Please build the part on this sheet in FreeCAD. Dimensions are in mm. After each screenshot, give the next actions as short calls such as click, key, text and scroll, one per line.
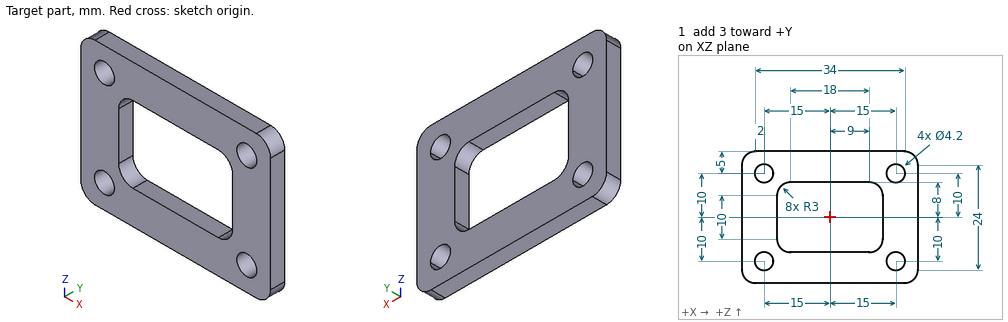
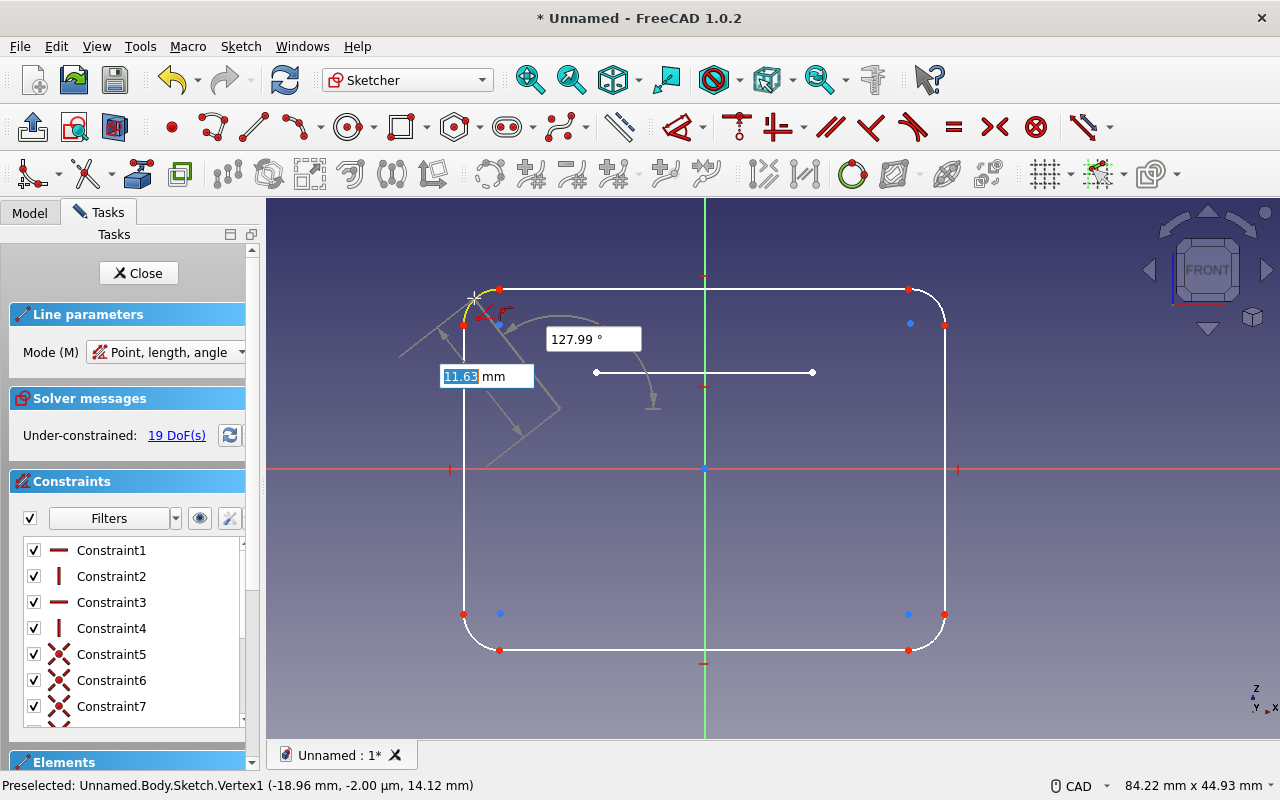
click(560, 529)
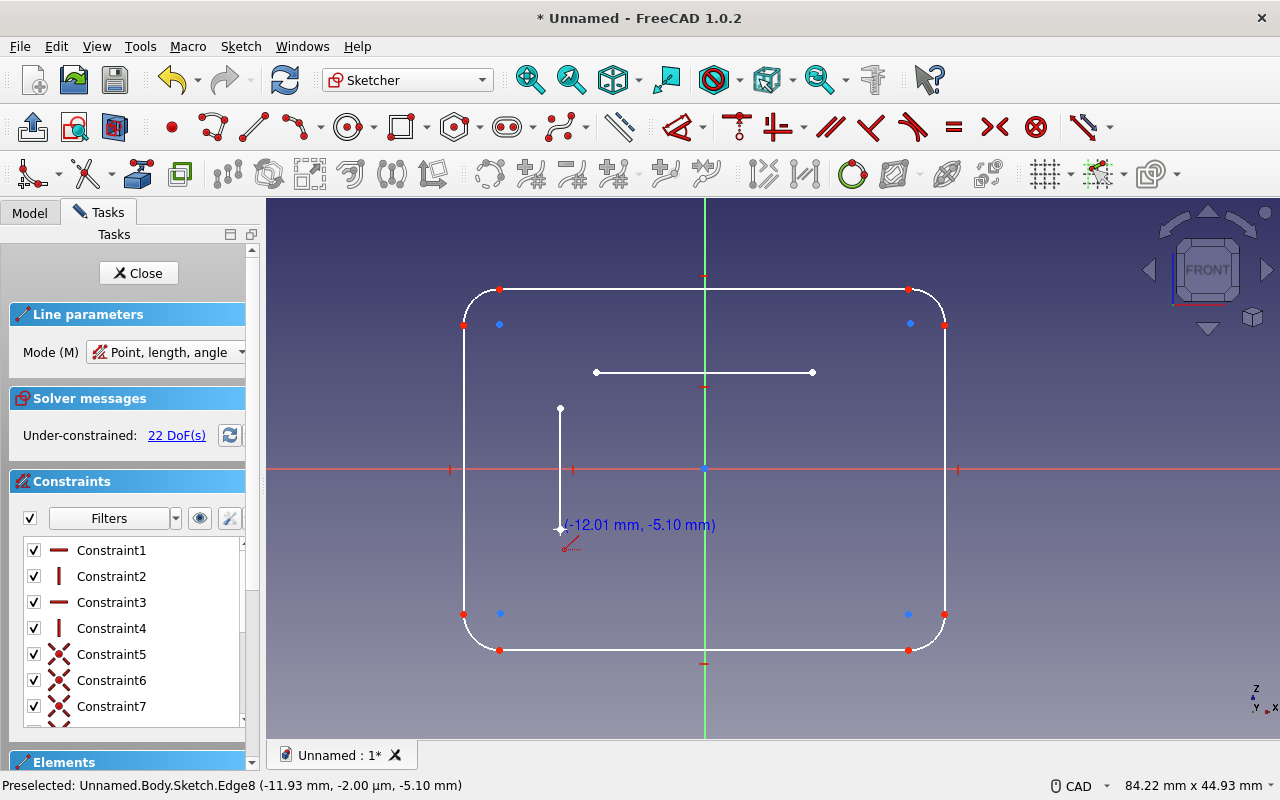
click(596, 565)
click(813, 565)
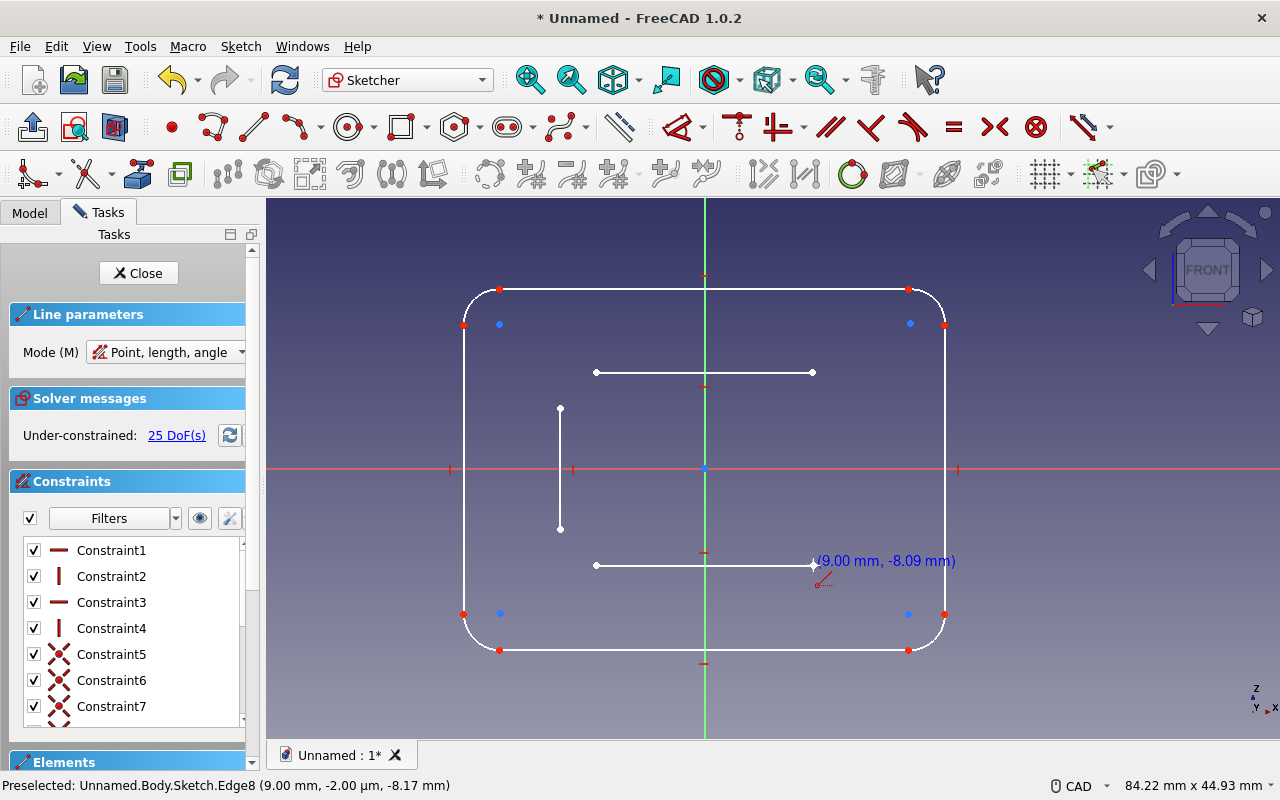
click(849, 529)
click(849, 408)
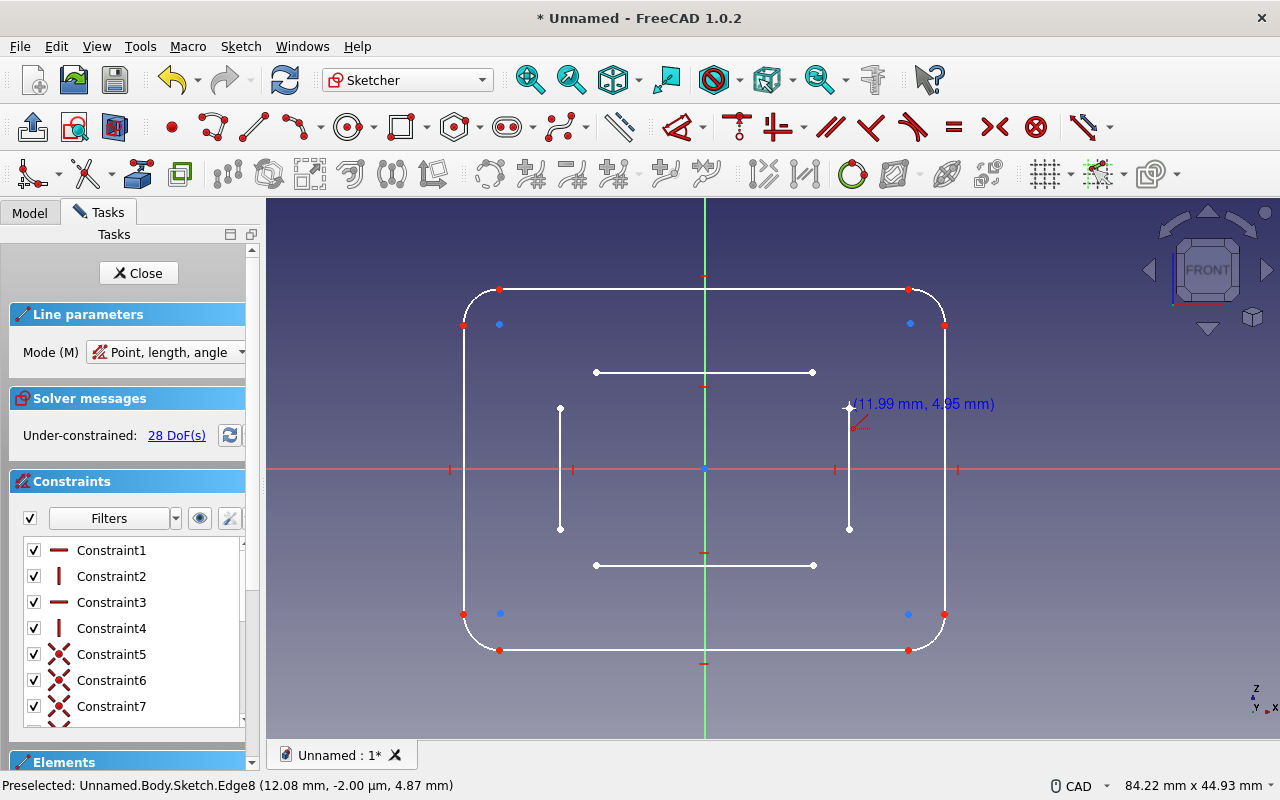
key(g)
key(3)
key(a)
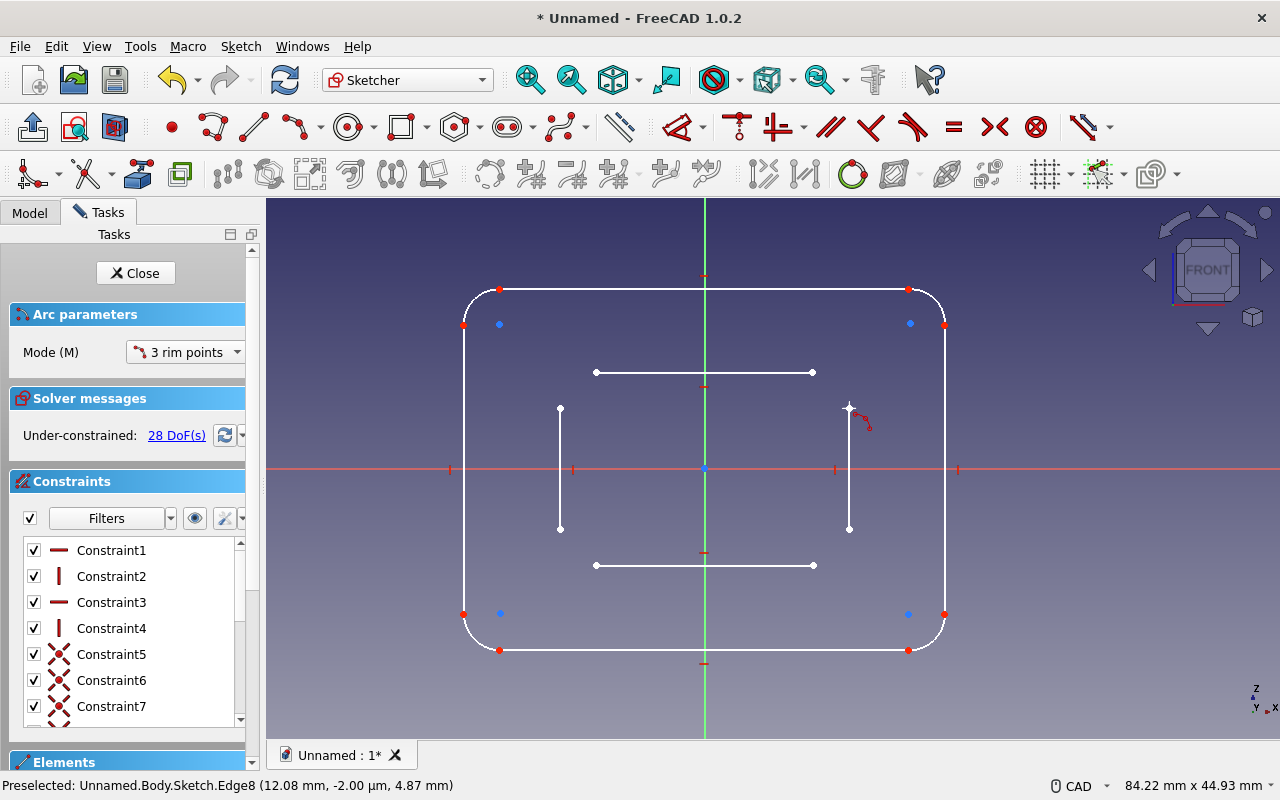
click(596, 373)
click(560, 409)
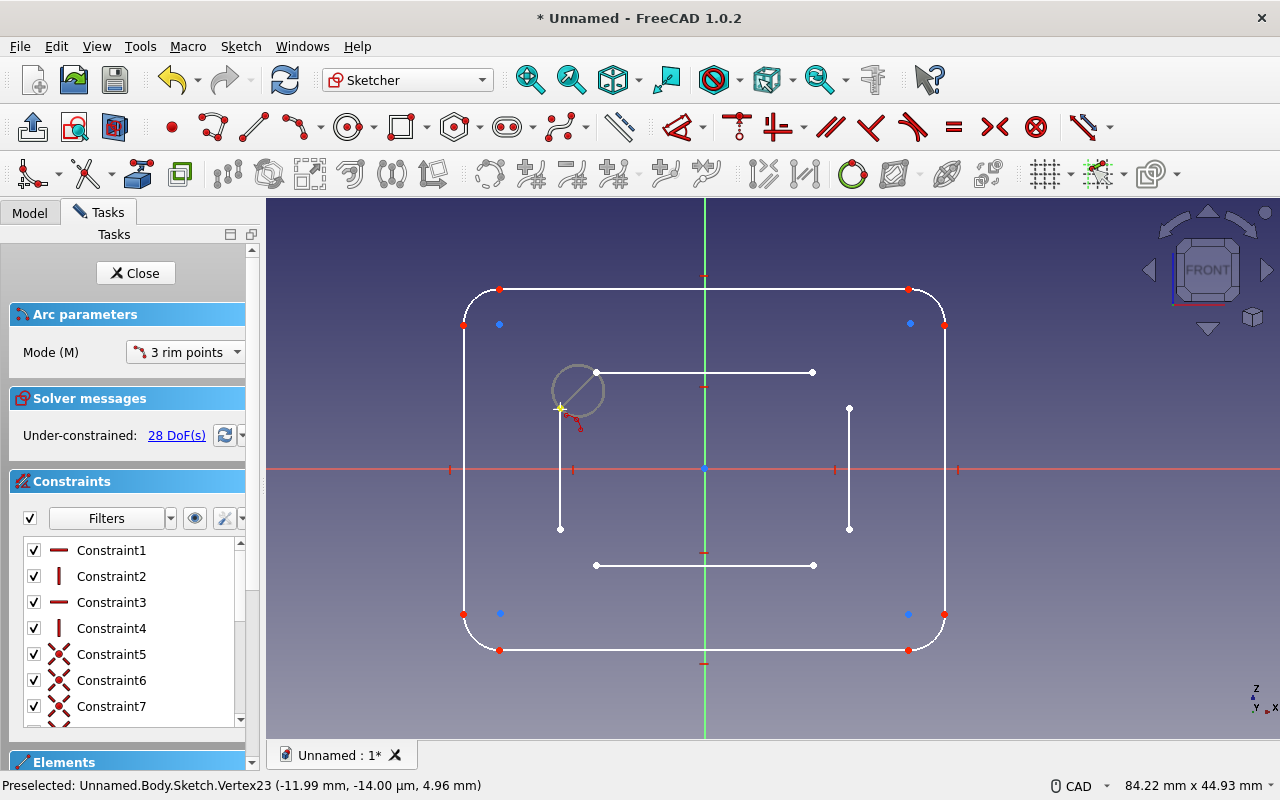
scroll(571, 383, up, 3)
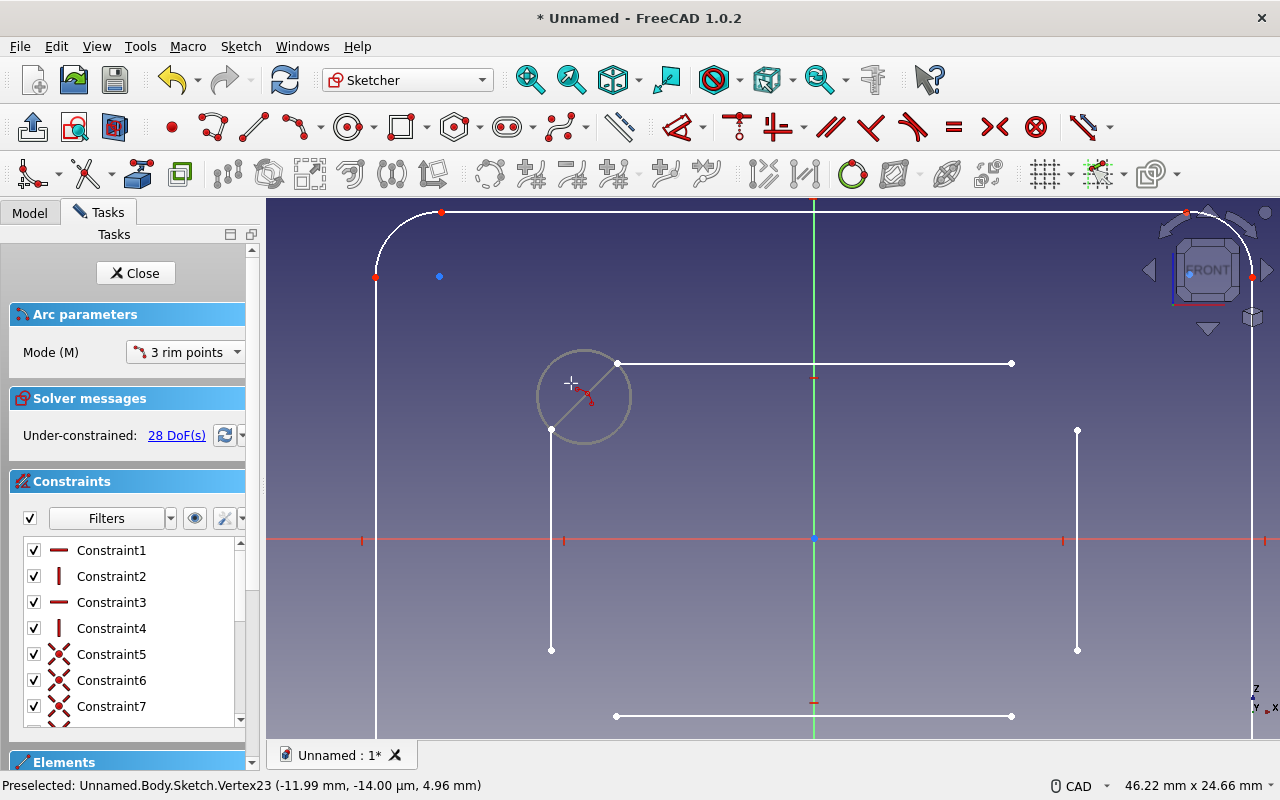
click(570, 383)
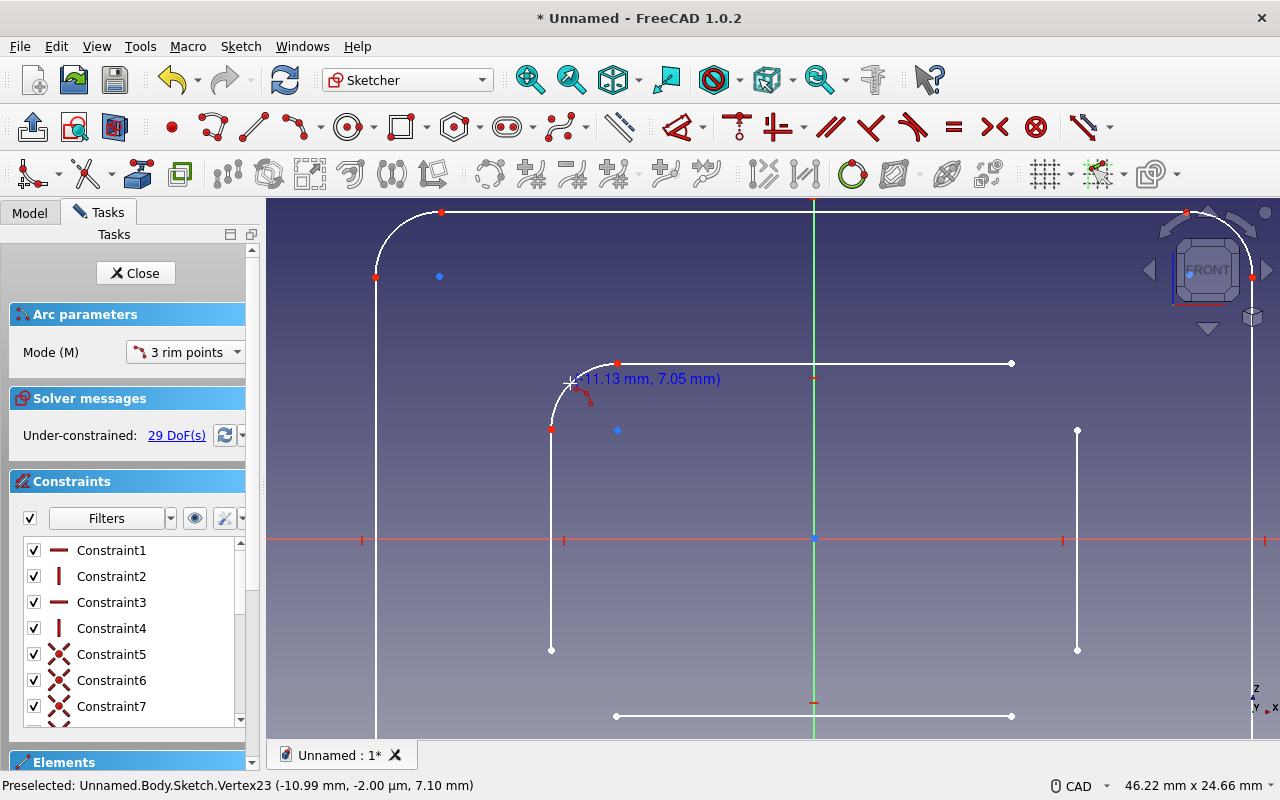
click(551, 651)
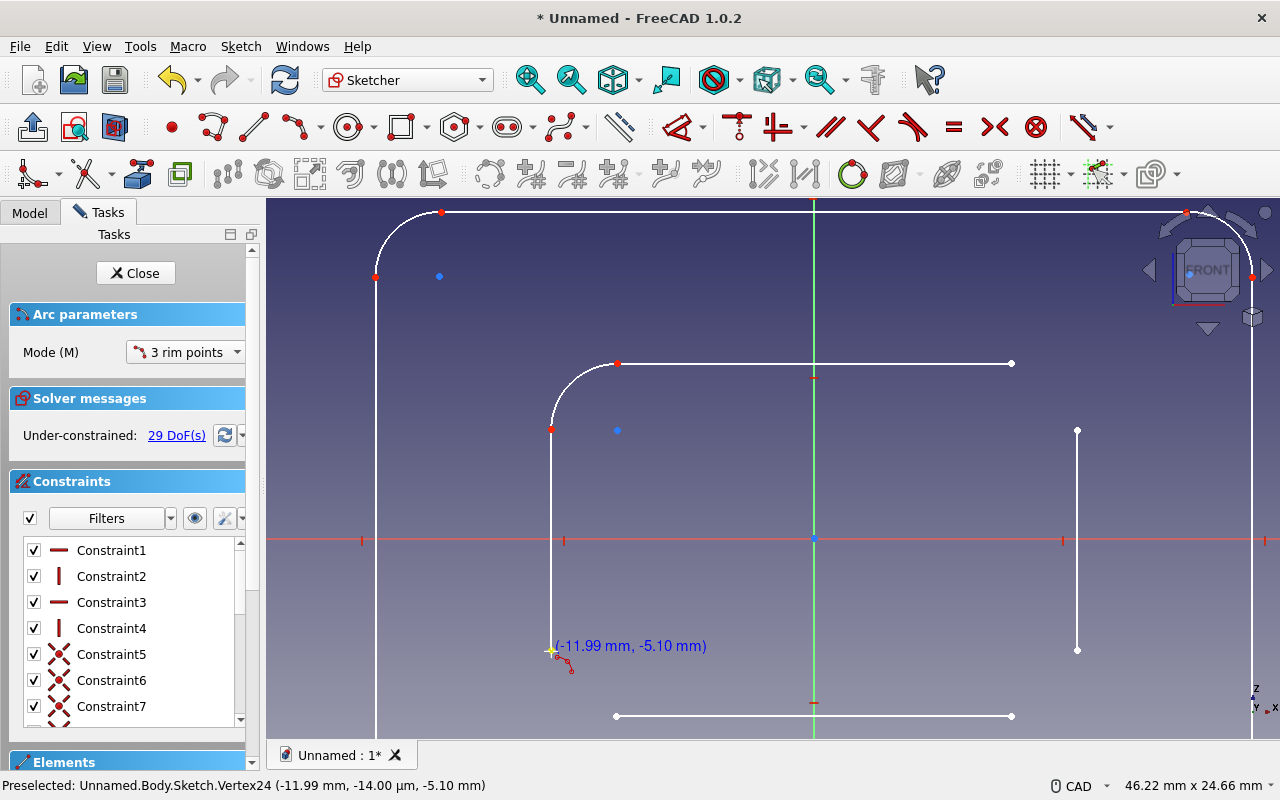
scroll(571, 383, down, 3)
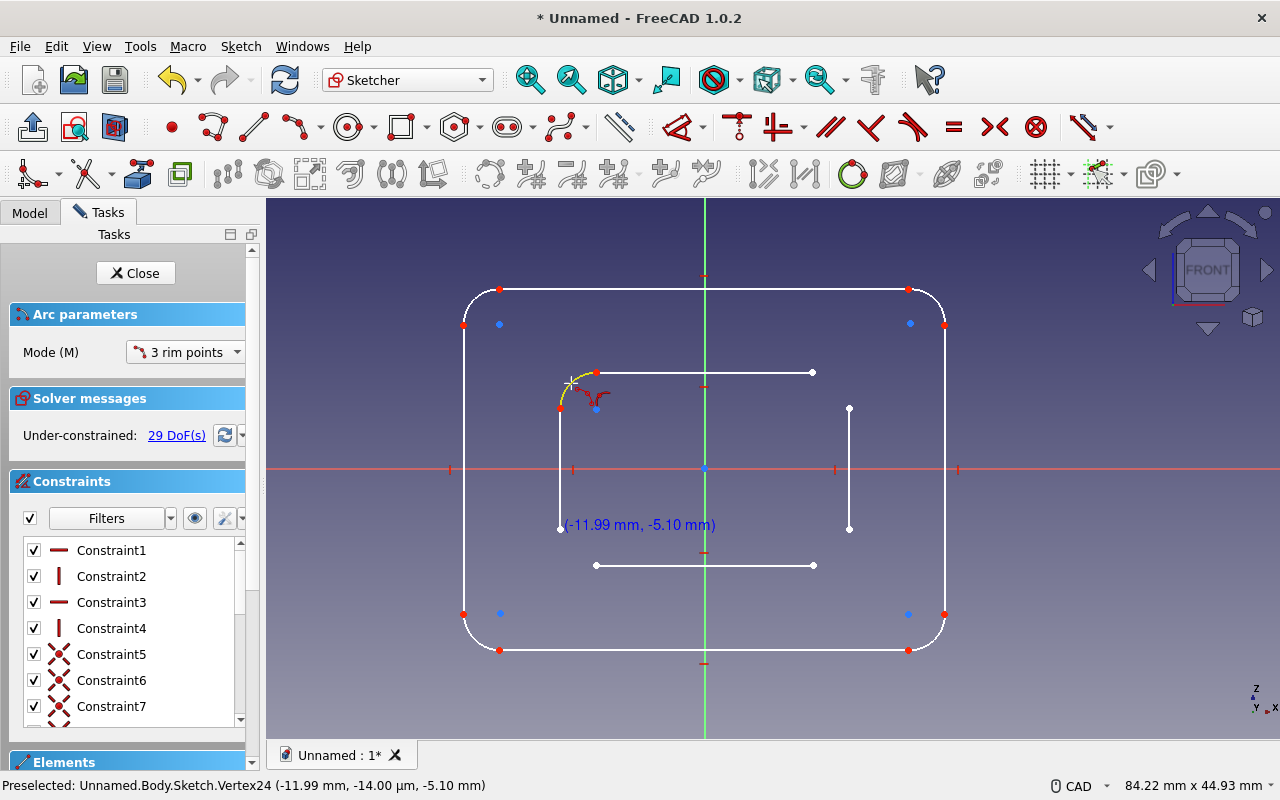
click(596, 566)